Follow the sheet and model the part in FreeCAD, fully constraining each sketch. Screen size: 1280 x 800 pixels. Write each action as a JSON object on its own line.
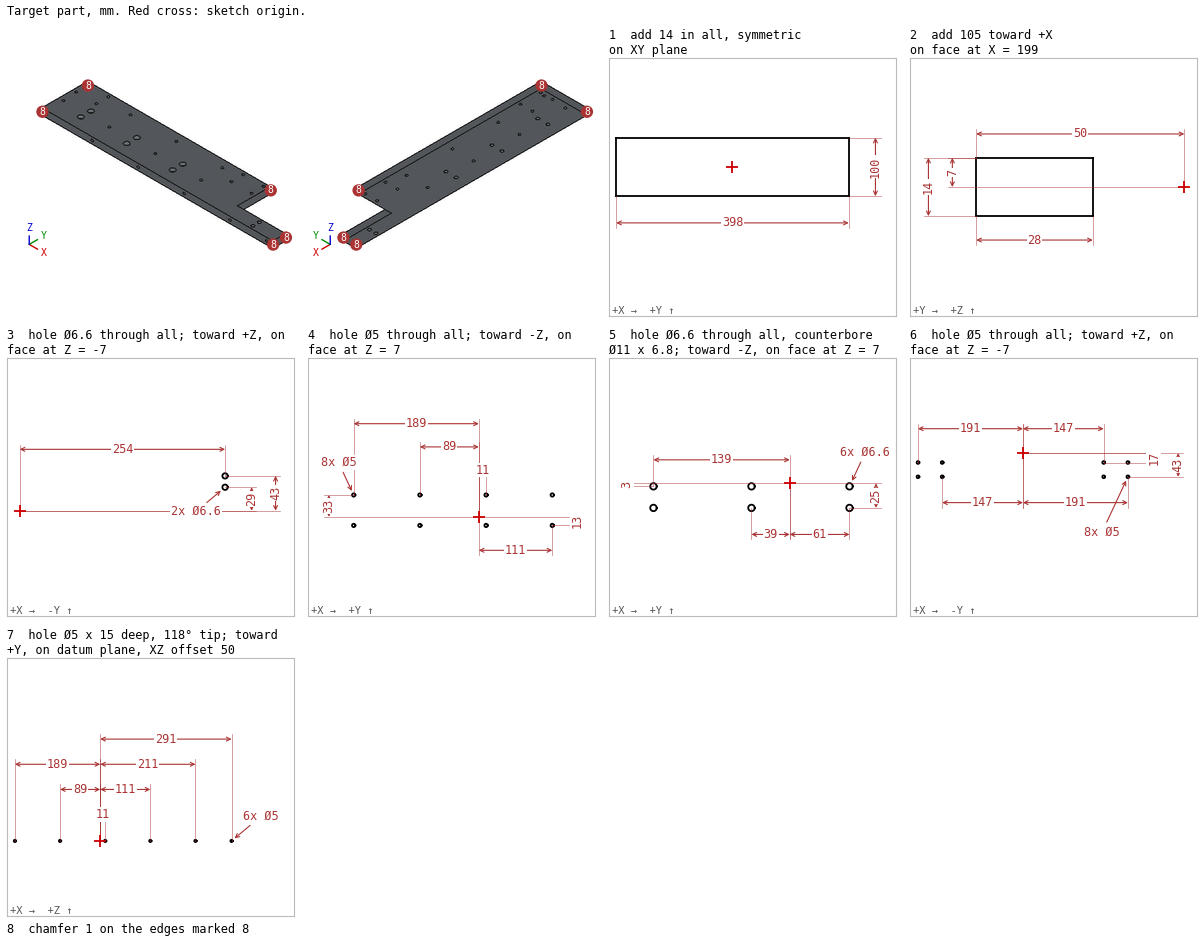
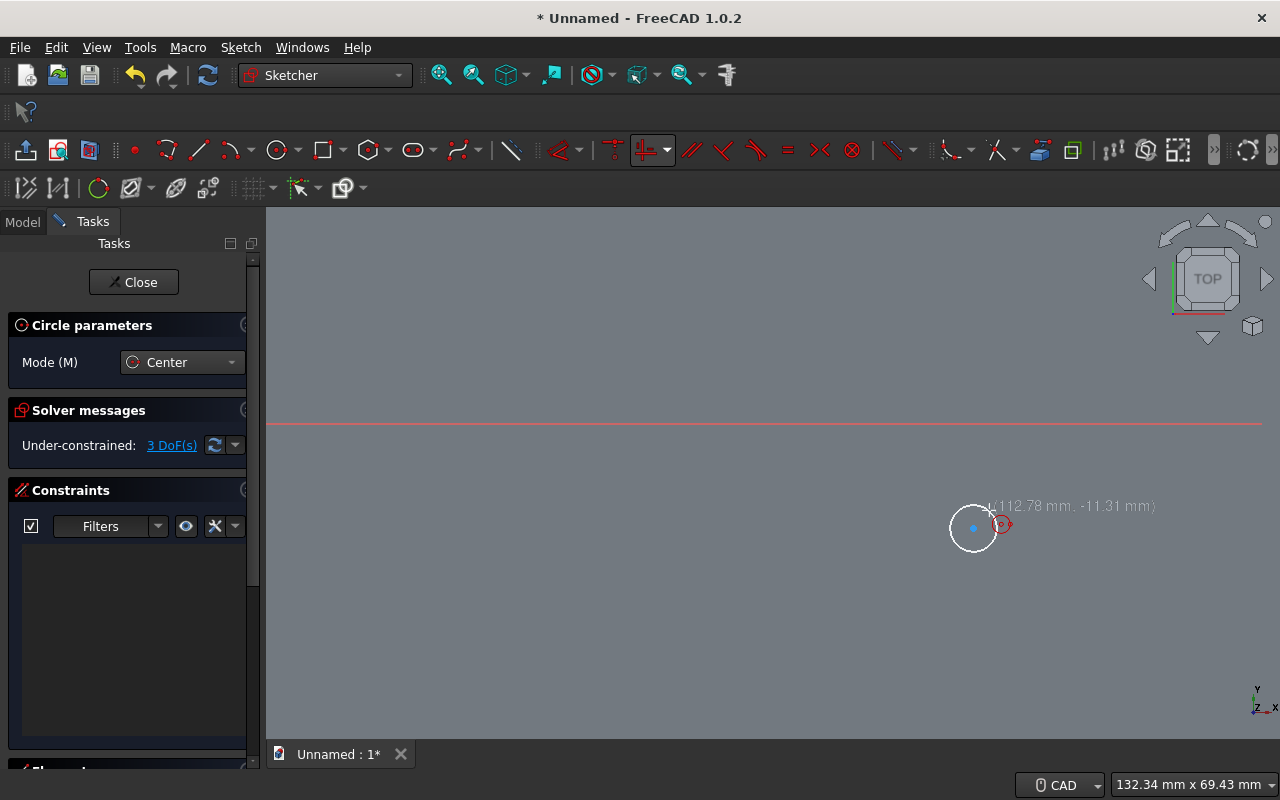
{"action": "scroll", "coordinate": [992, 514], "scroll_direction": "down", "scroll_amount": 7}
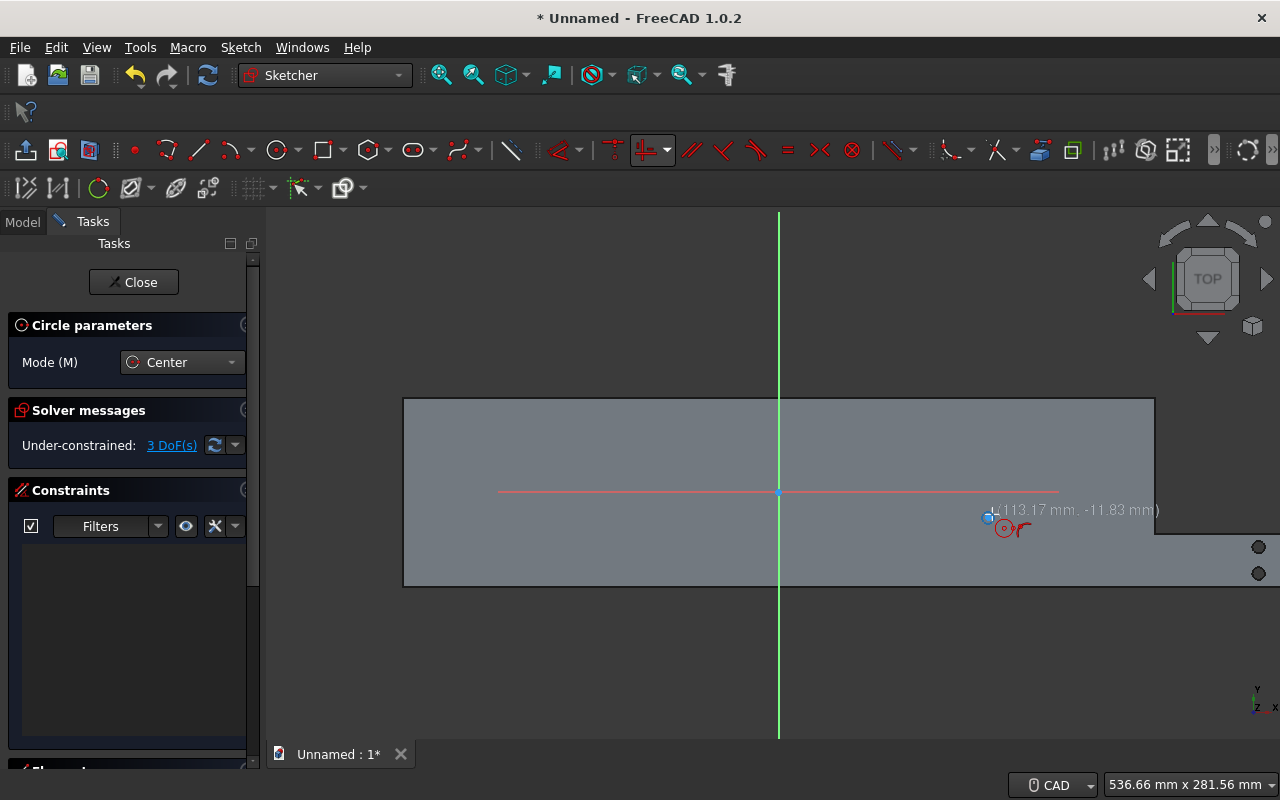
{"action": "scroll", "coordinate": [422, 430], "scroll_direction": "up", "scroll_amount": 8}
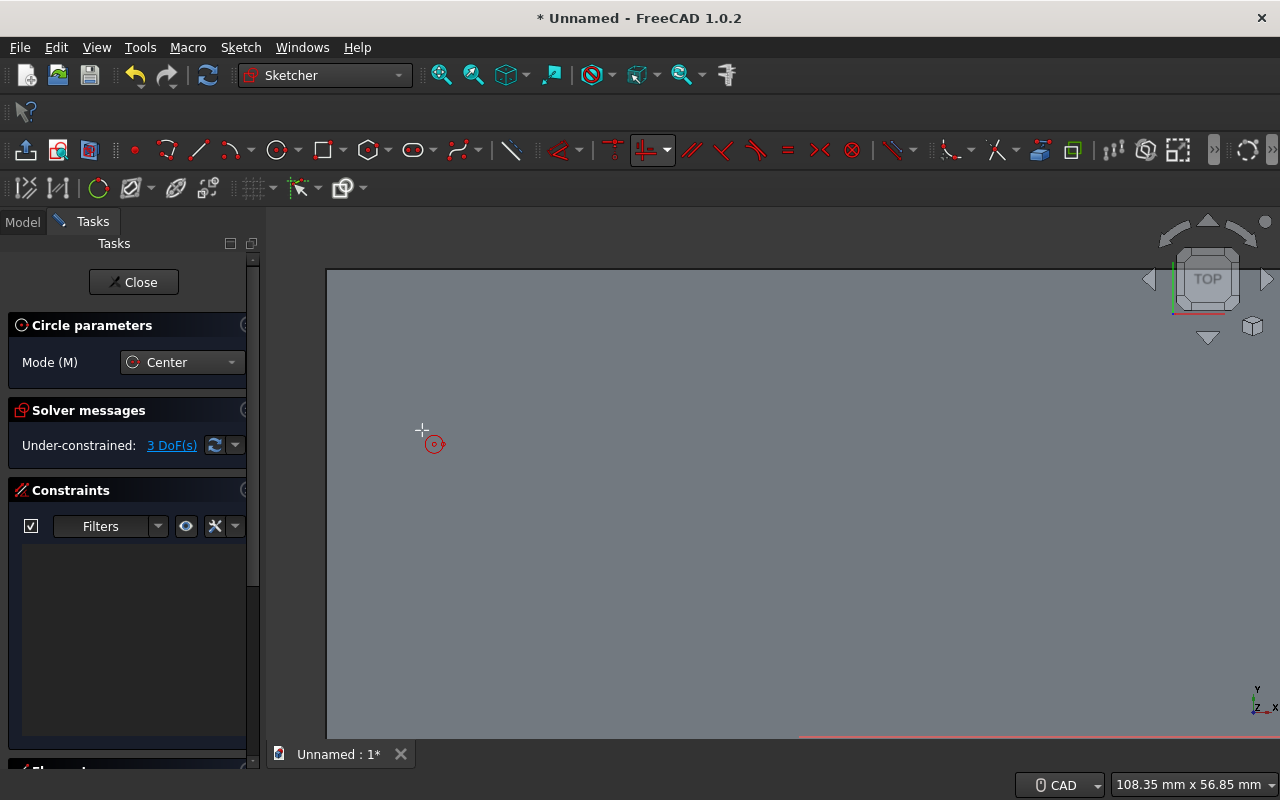
{"action": "scroll", "coordinate": [422, 430], "scroll_direction": "down", "scroll_amount": 8}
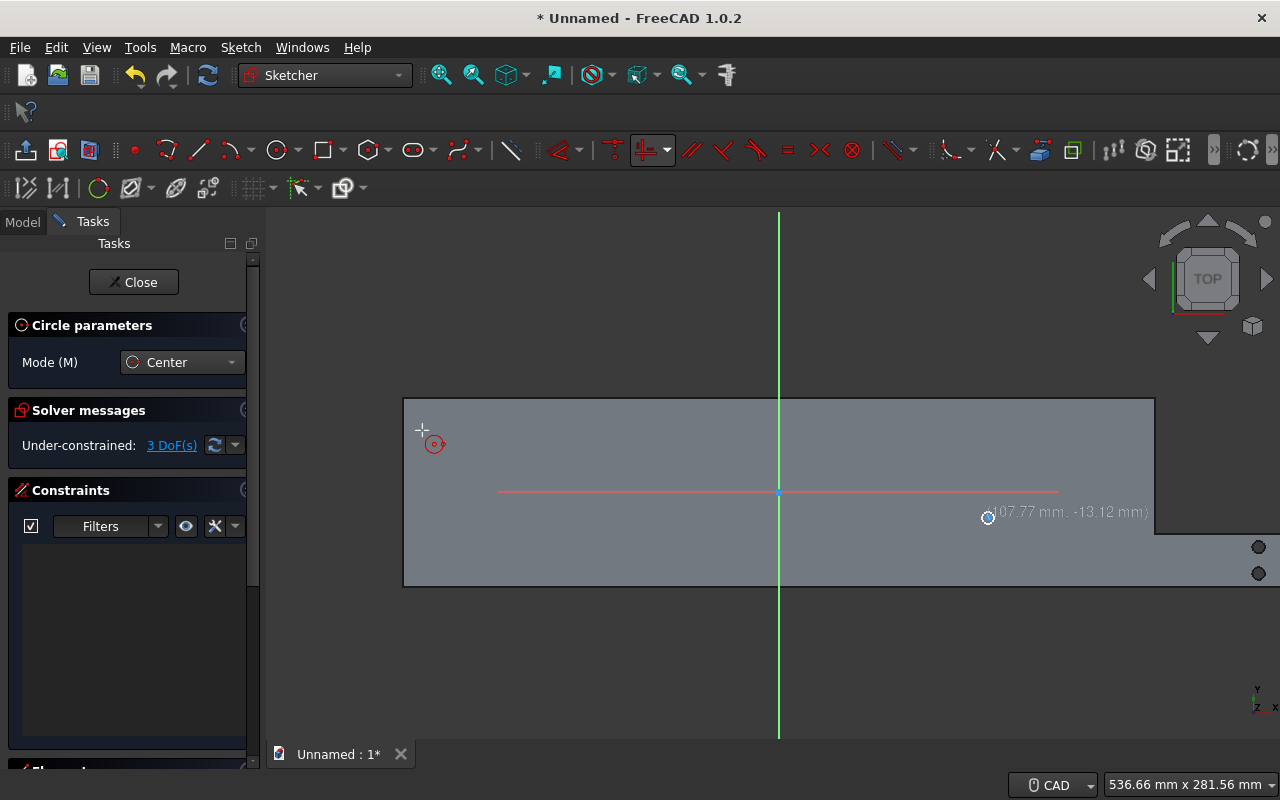
{"action": "left_click", "coordinate": [422, 430]}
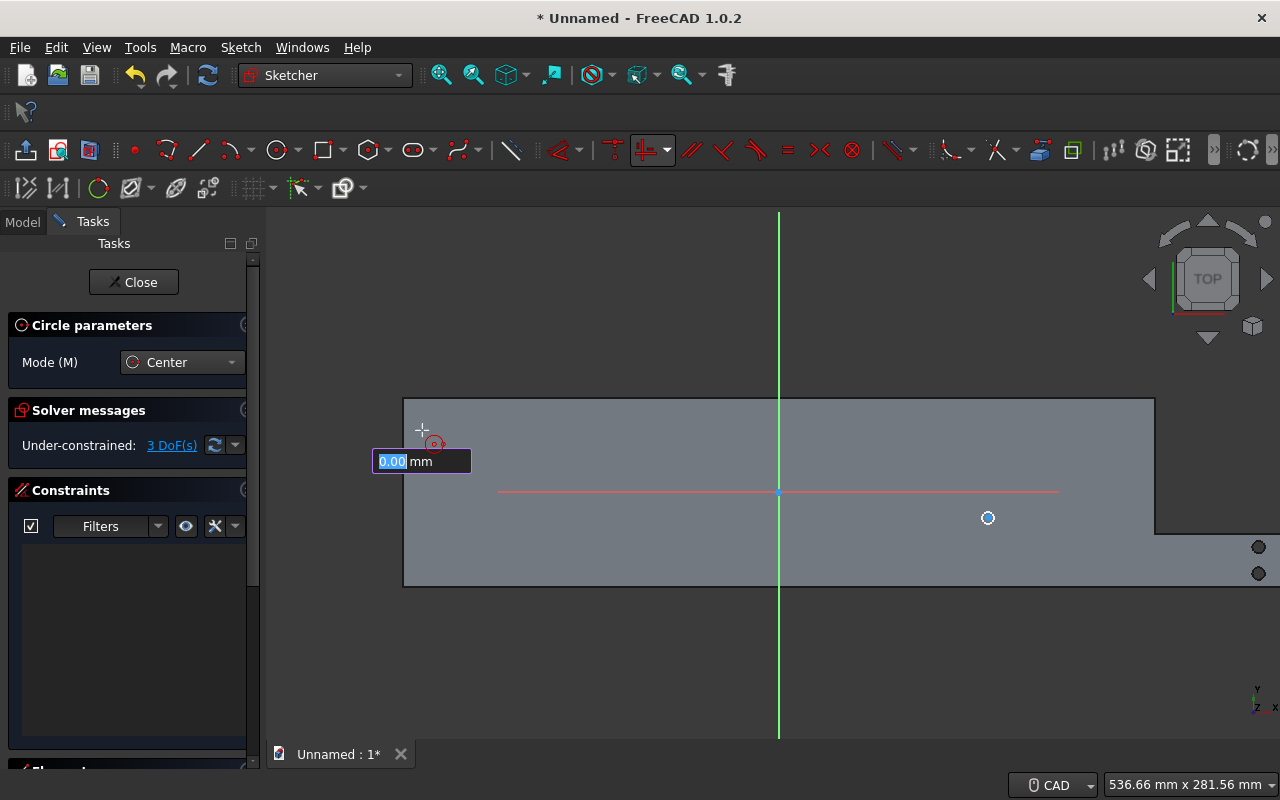
{"action": "scroll", "coordinate": [425, 427], "scroll_direction": "up", "scroll_amount": 7}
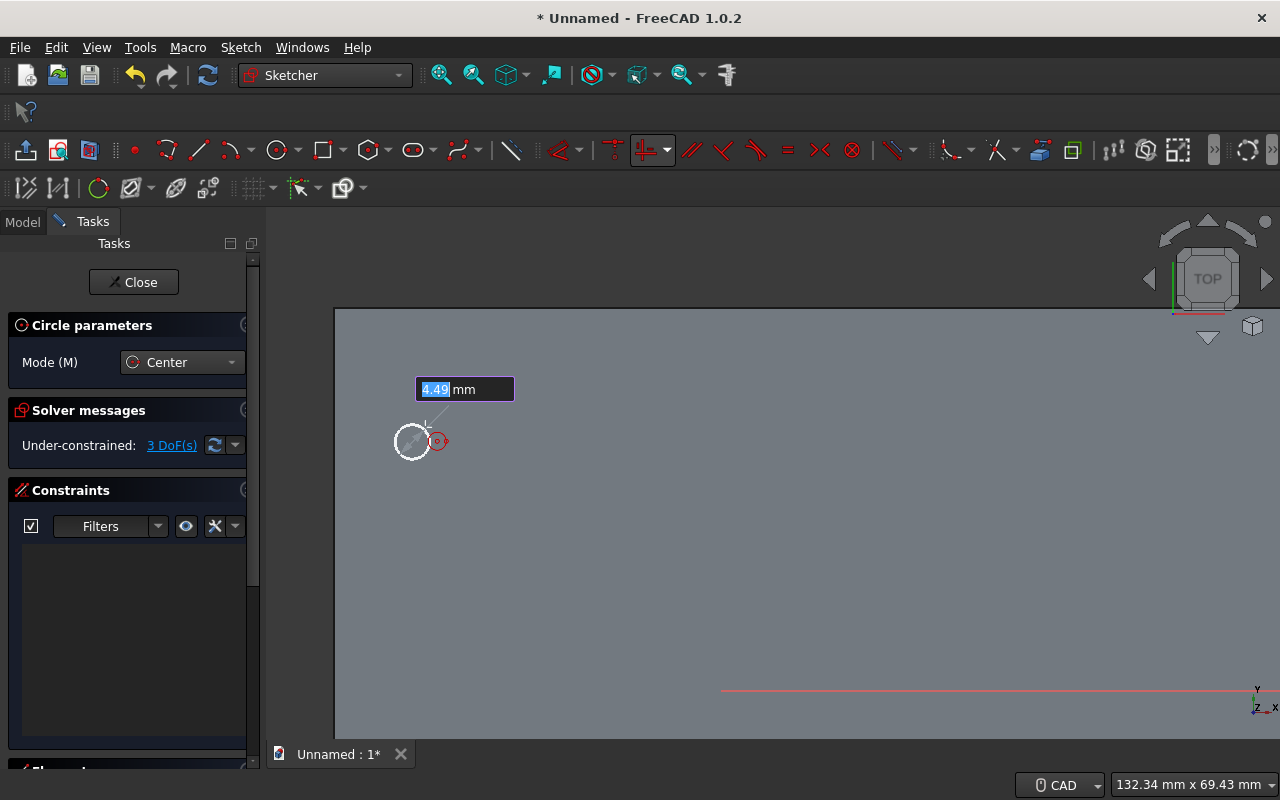
{"action": "left_click", "coordinate": [424, 424]}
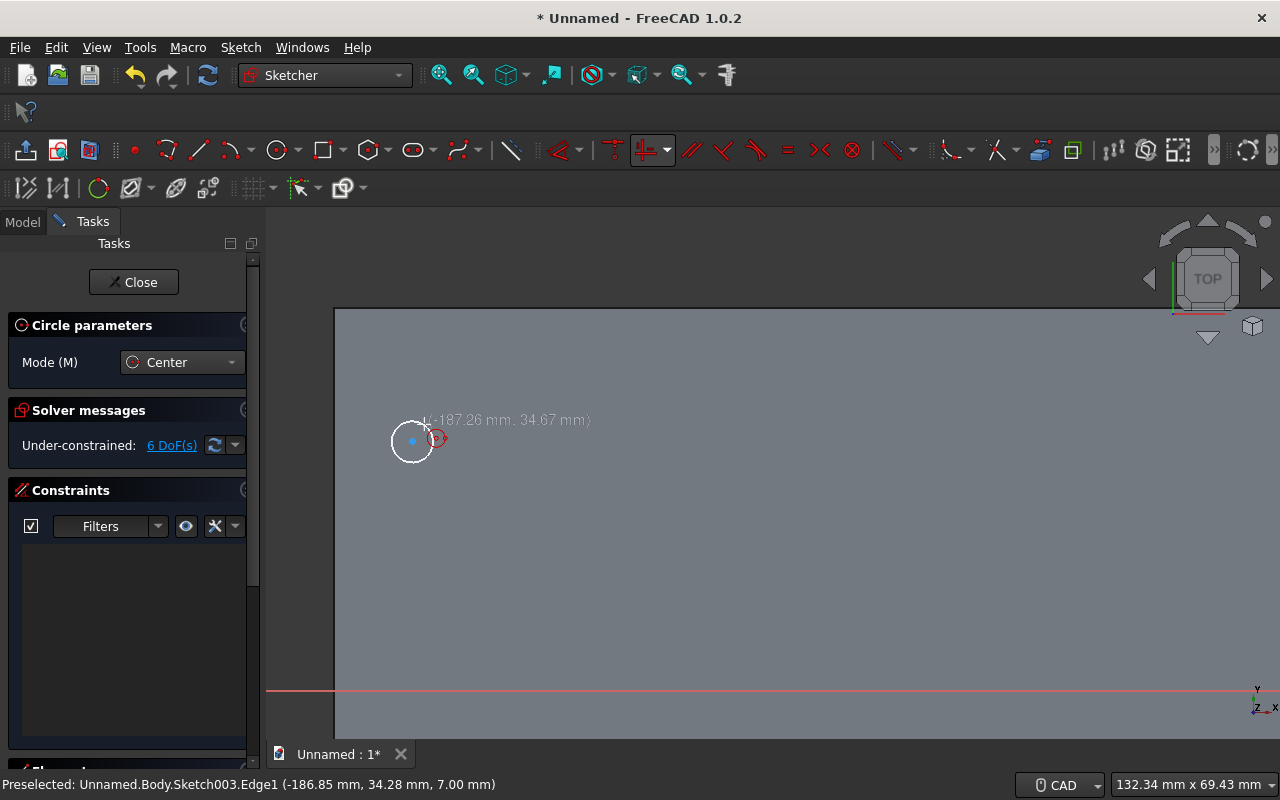
{"action": "scroll", "coordinate": [424, 427], "scroll_direction": "down", "scroll_amount": 7}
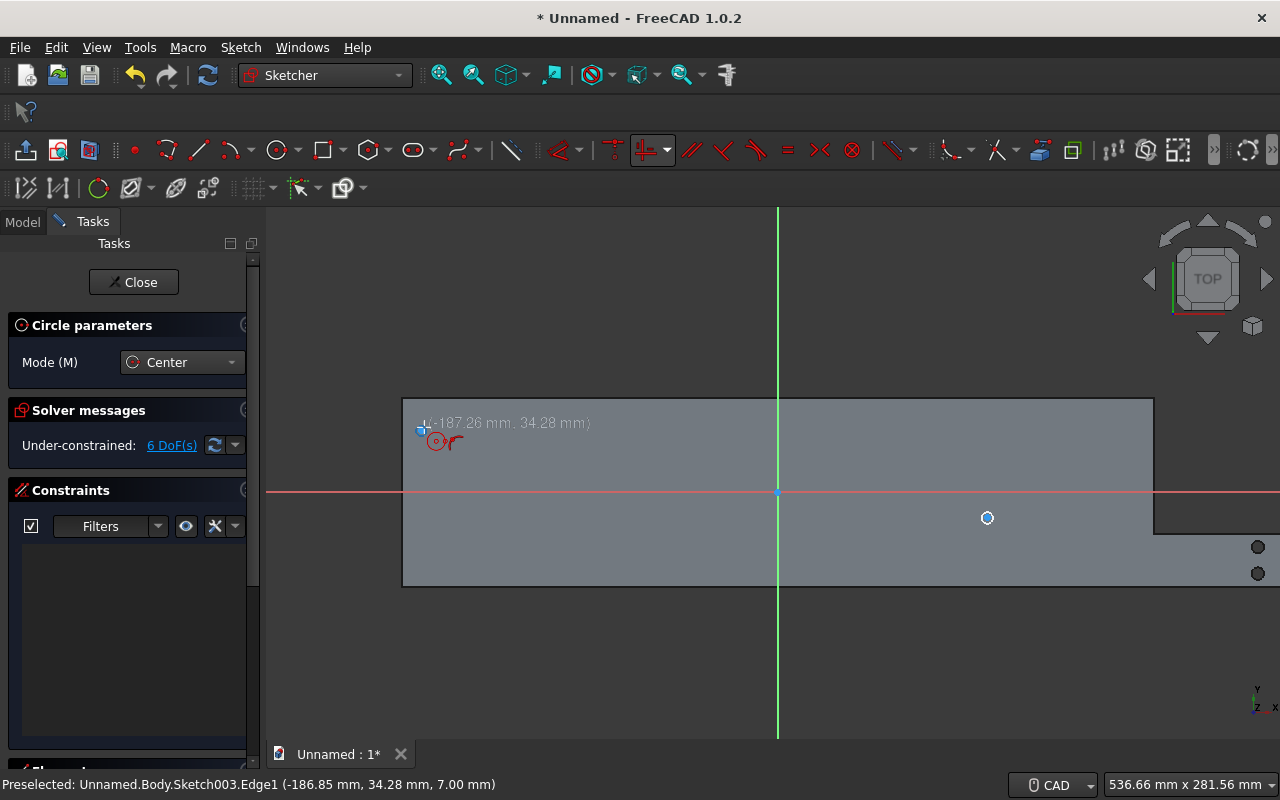
{"action": "scroll", "coordinate": [421, 517], "scroll_direction": "up", "scroll_amount": 8}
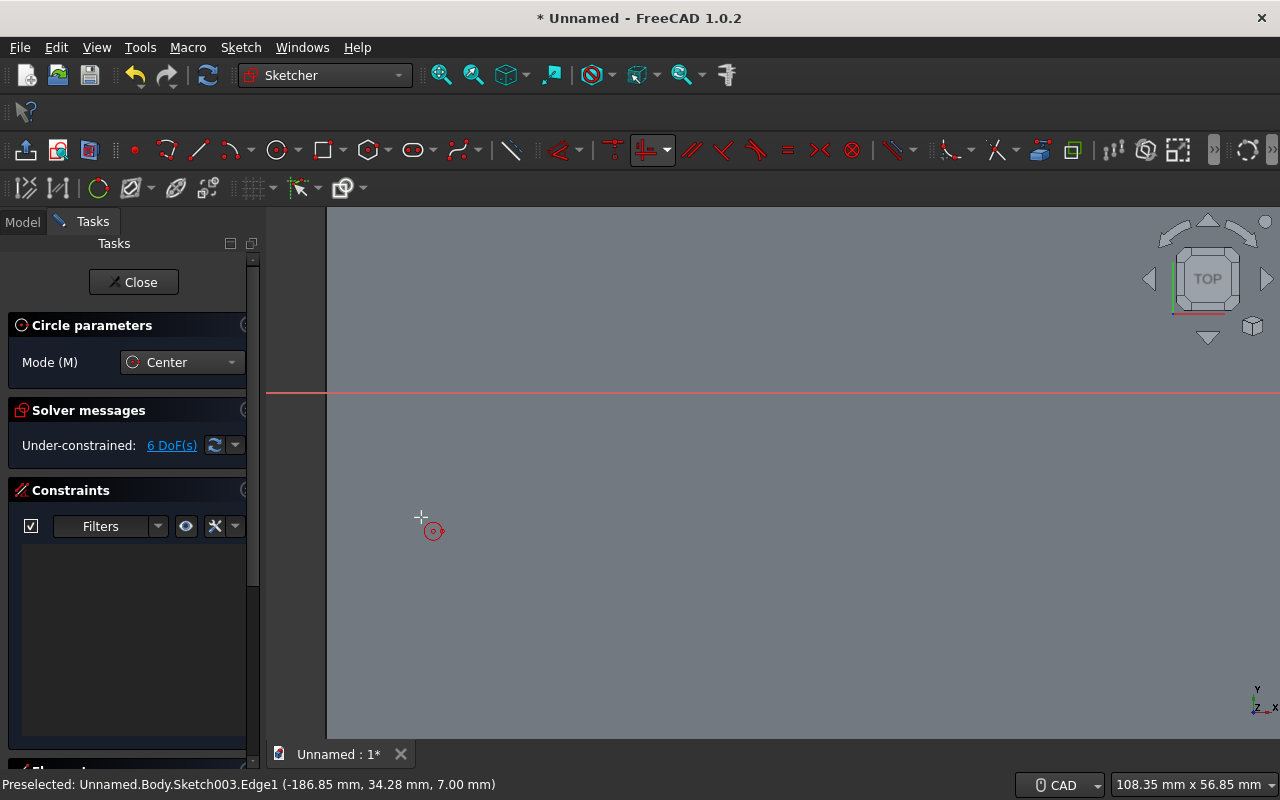
{"action": "scroll", "coordinate": [421, 517], "scroll_direction": "down", "scroll_amount": 8}